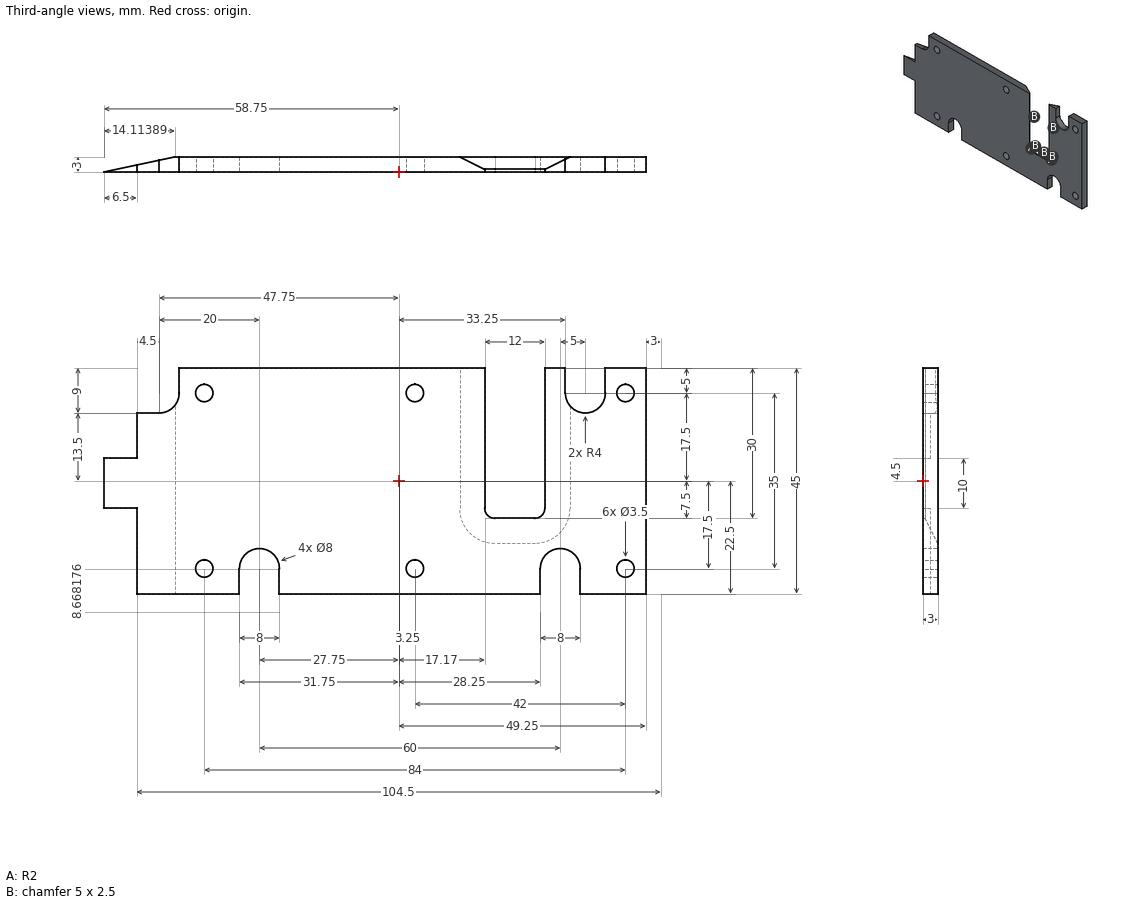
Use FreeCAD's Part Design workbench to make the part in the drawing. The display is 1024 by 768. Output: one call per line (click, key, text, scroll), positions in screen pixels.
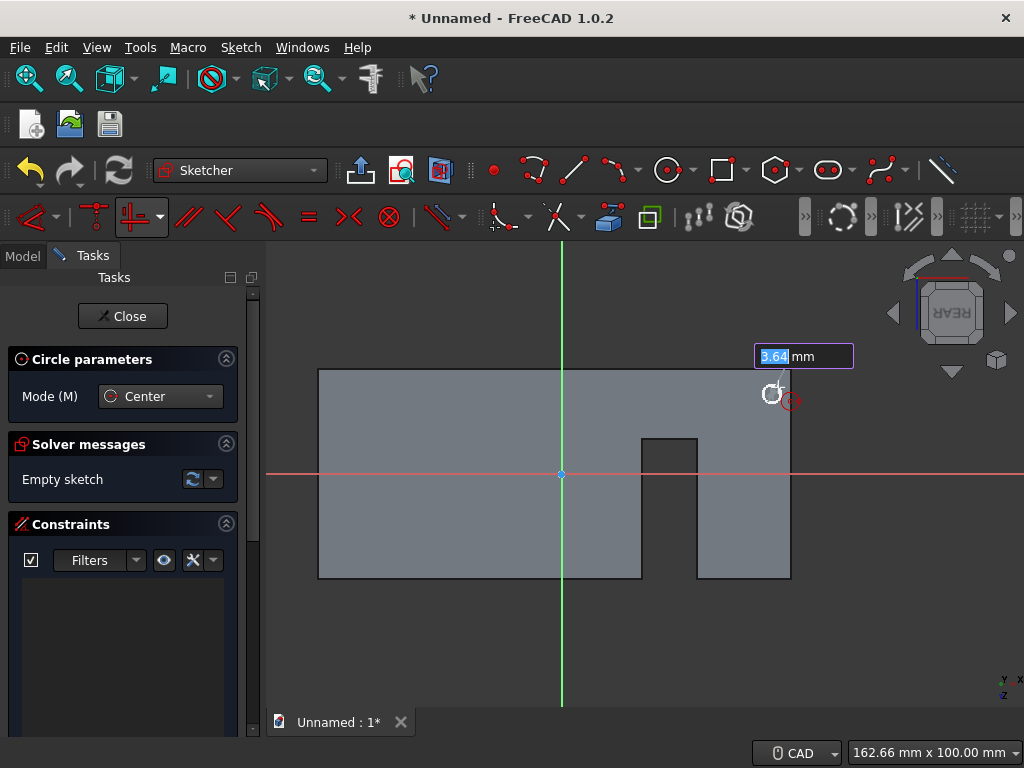
text(3.5)
key(Return)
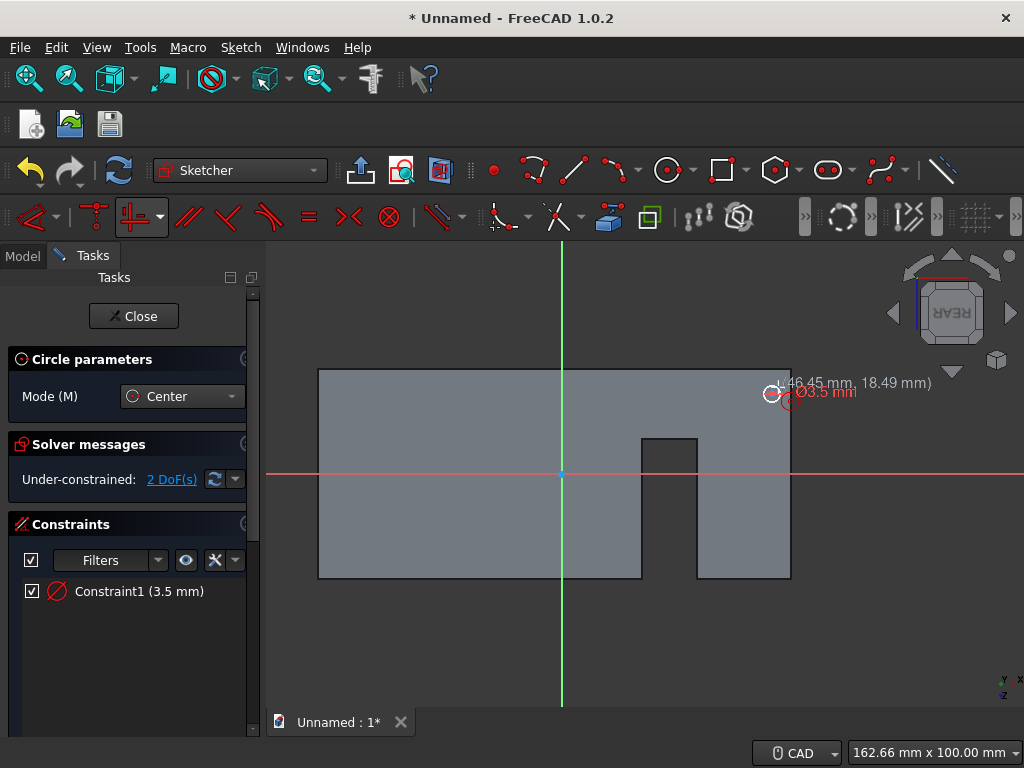
scroll(772, 556, up, 6)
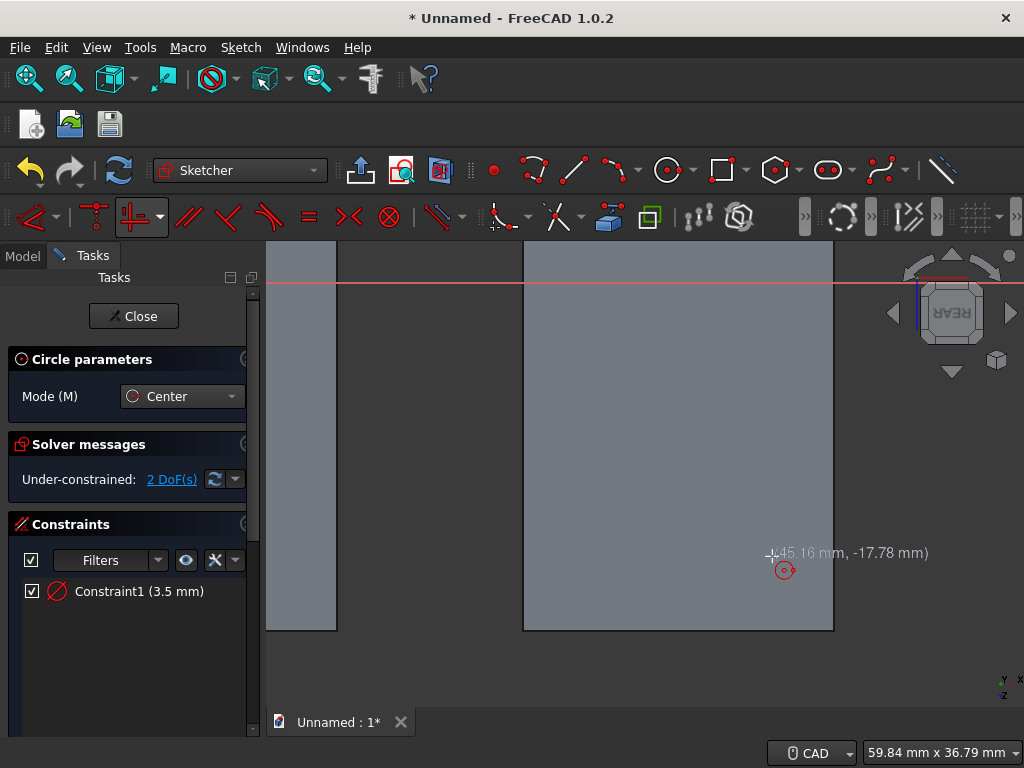
scroll(772, 556, down, 6)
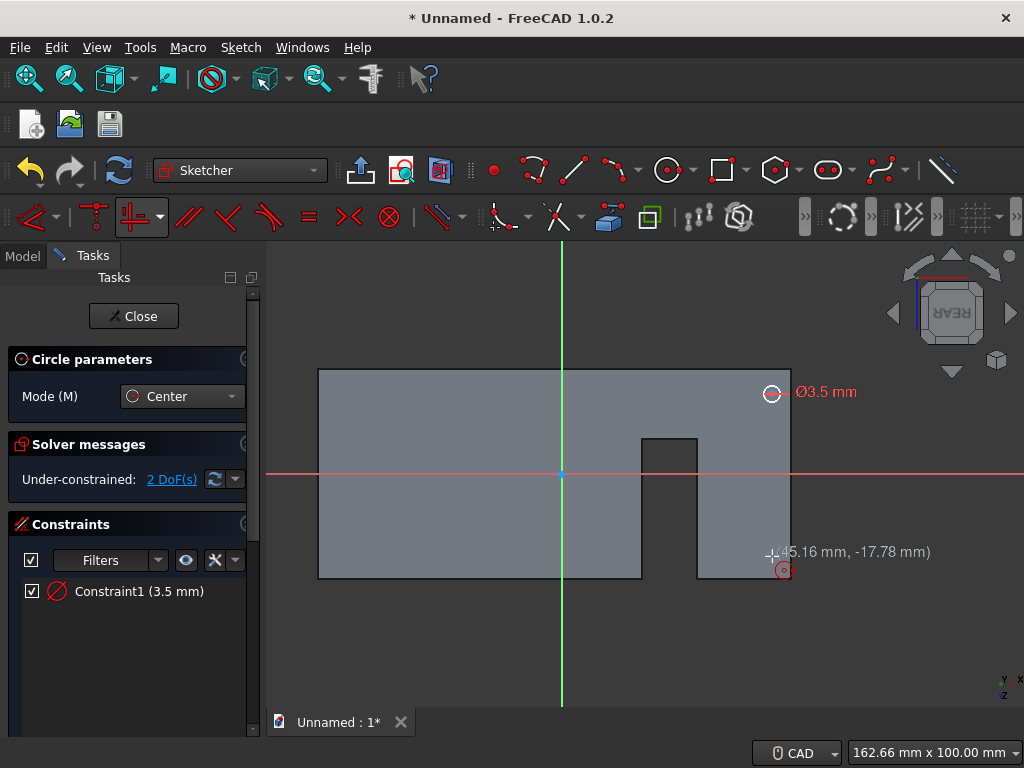
click(772, 556)
move(778, 550)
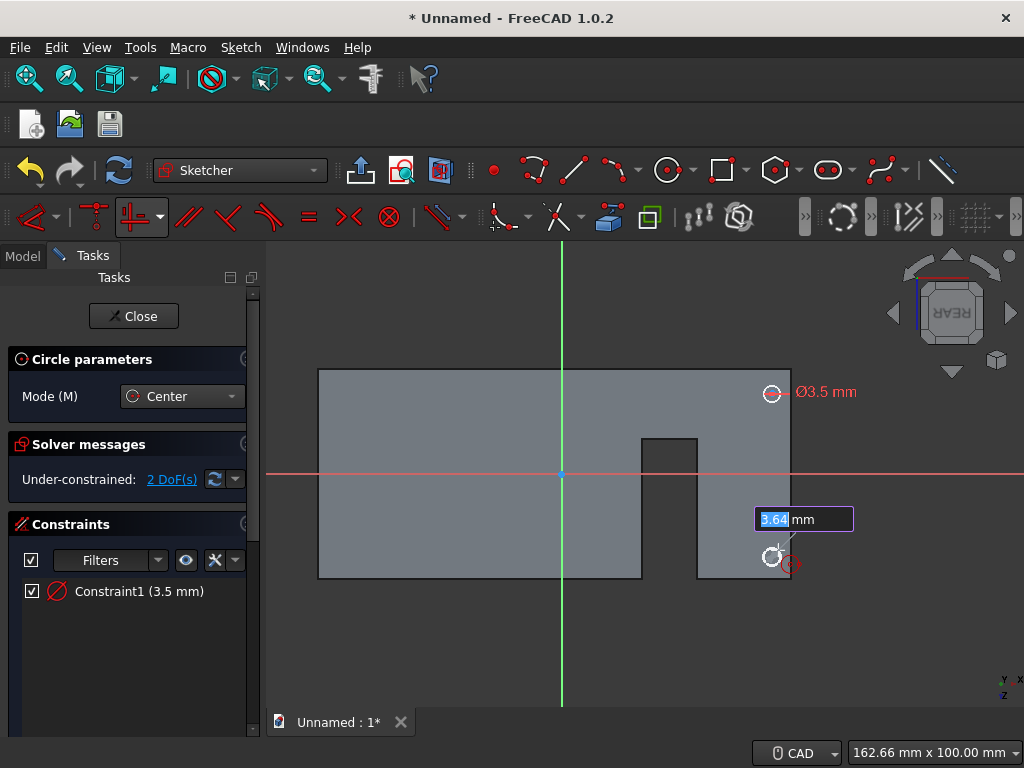
text(3.5)
key(Return)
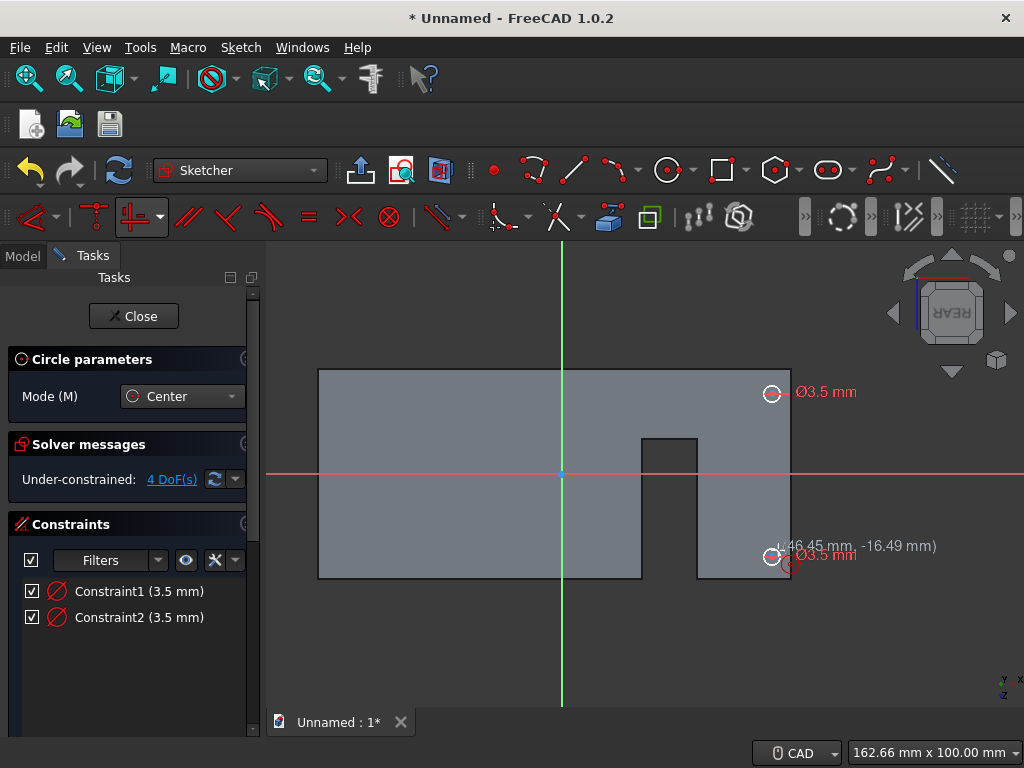
scroll(381, 393, up, 6)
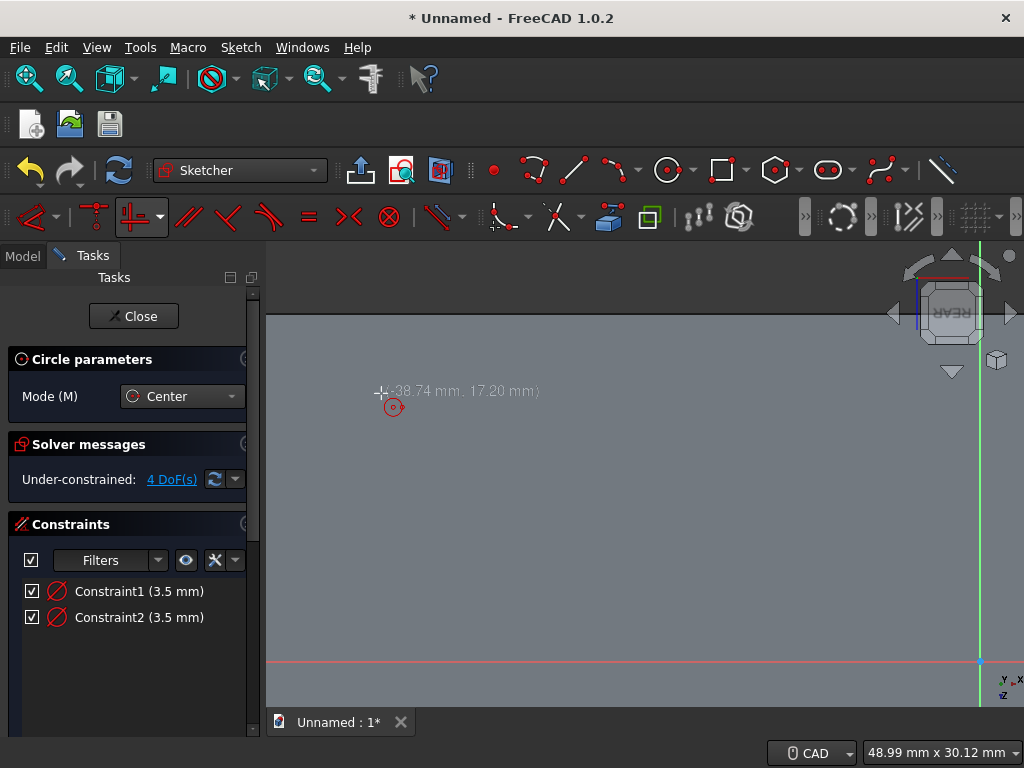
scroll(381, 393, down, 6)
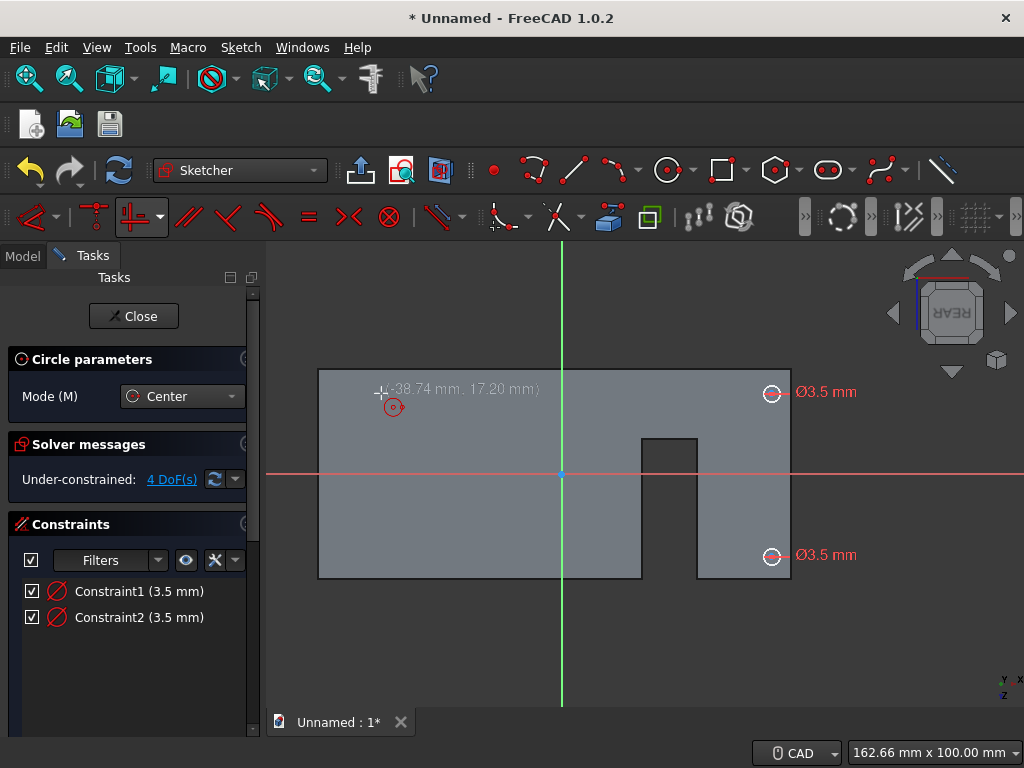
click(381, 393)
move(387, 387)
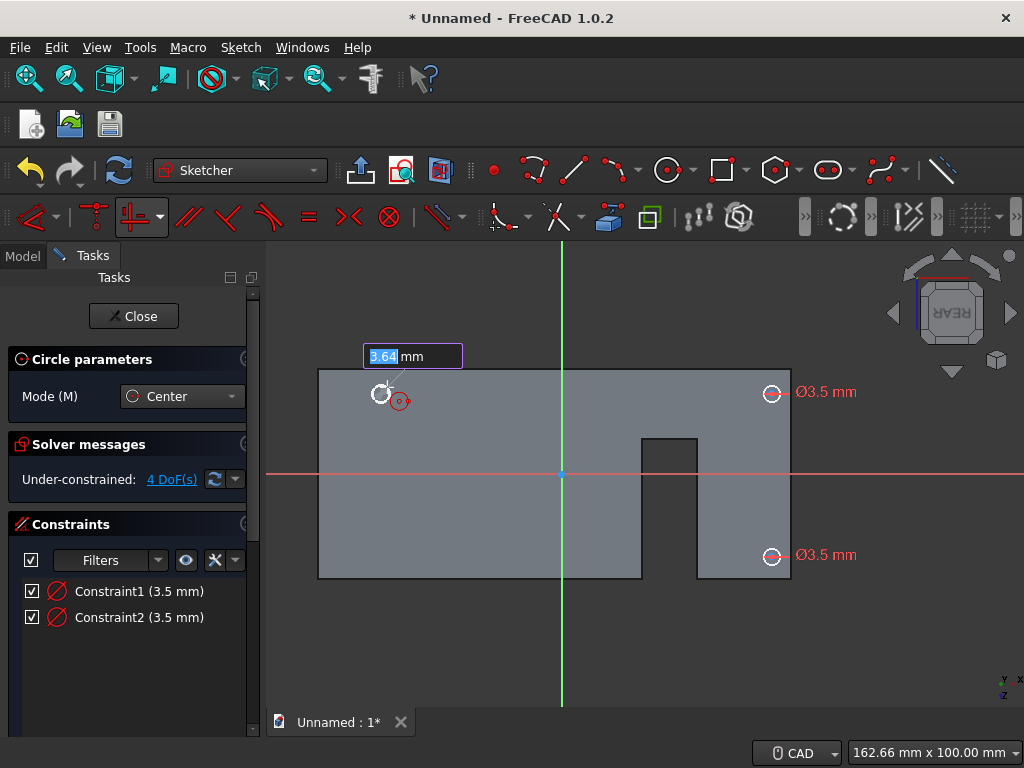
text(3.5)
key(Return)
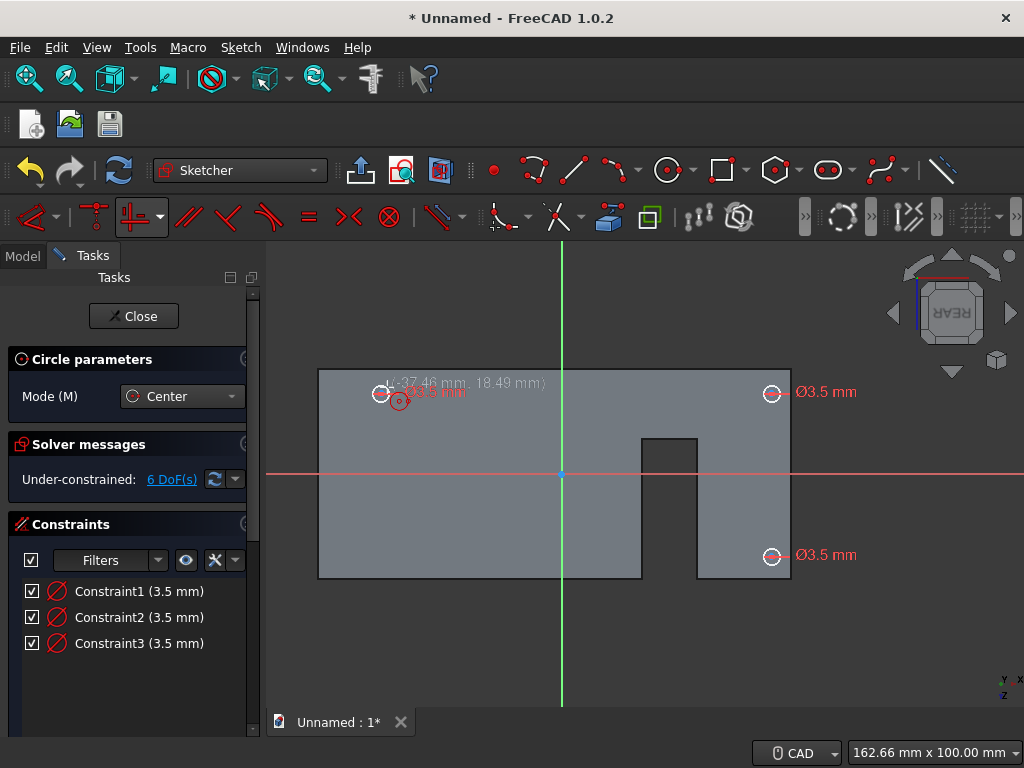
scroll(577, 393, up, 6)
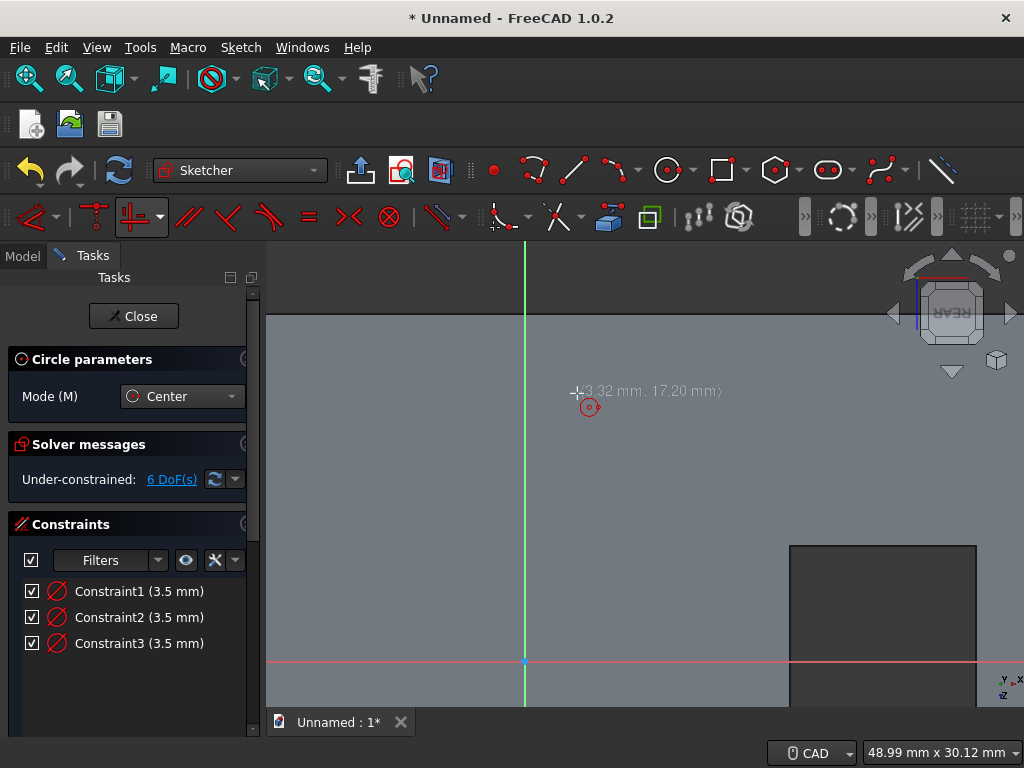
scroll(577, 393, down, 6)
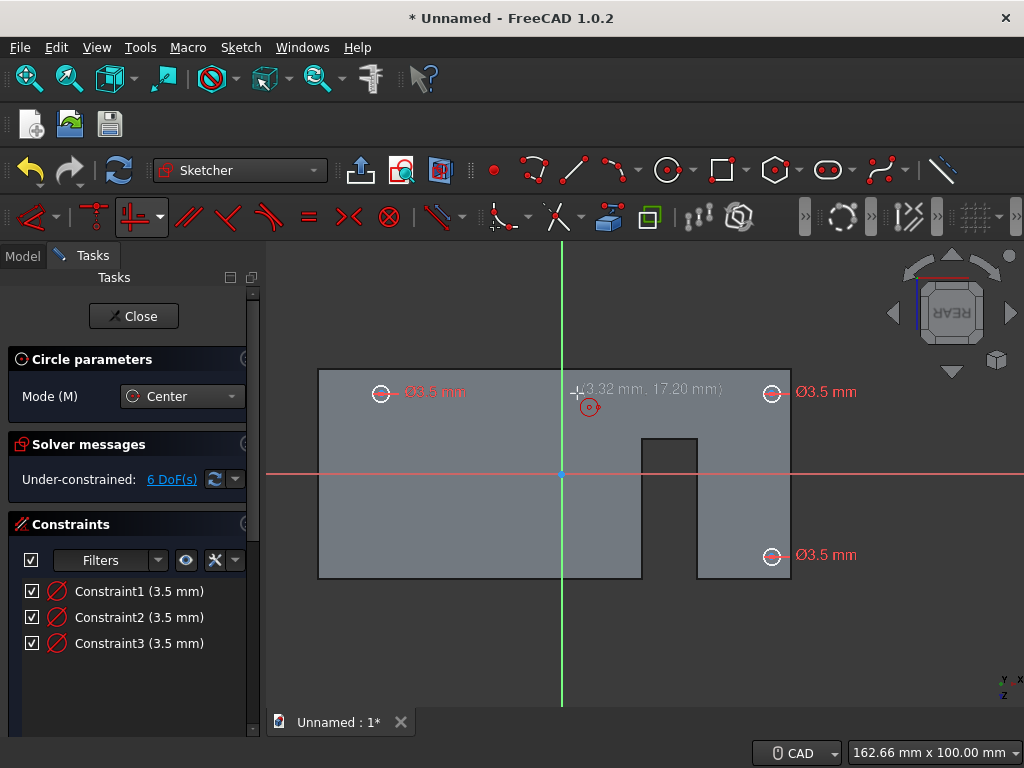
click(577, 393)
move(582, 387)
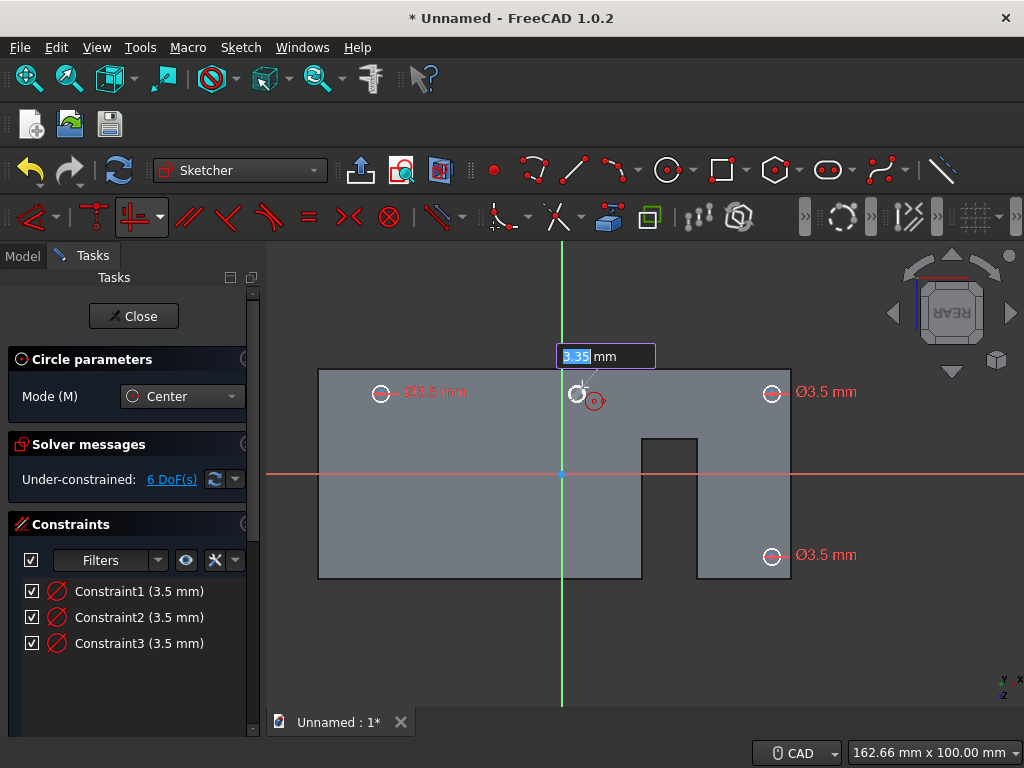
text(3.5)
key(Return)